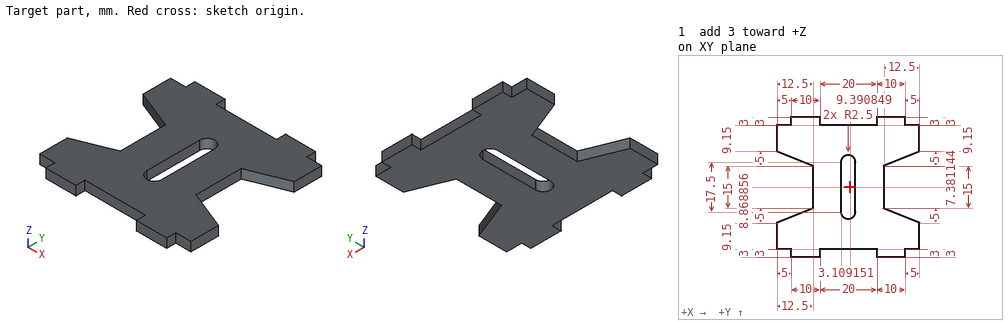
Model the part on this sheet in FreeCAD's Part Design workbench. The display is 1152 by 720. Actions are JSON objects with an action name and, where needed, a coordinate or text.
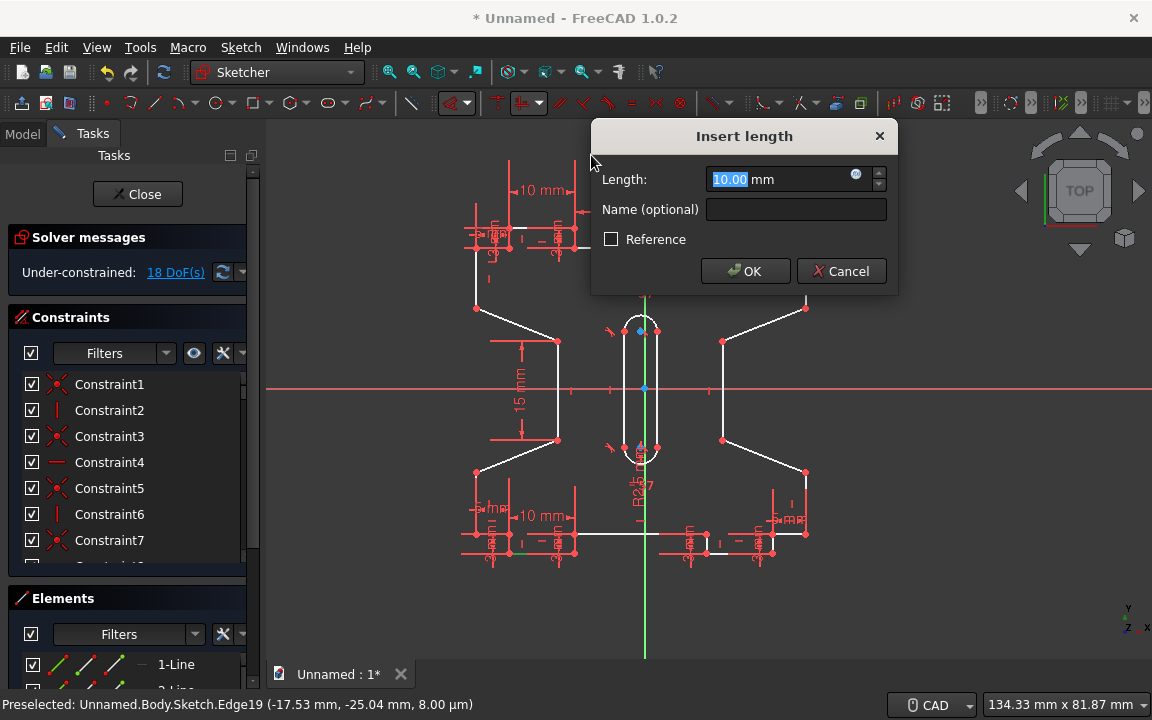
{"action": "type", "text": "10"}
{"action": "key", "text": "Return"}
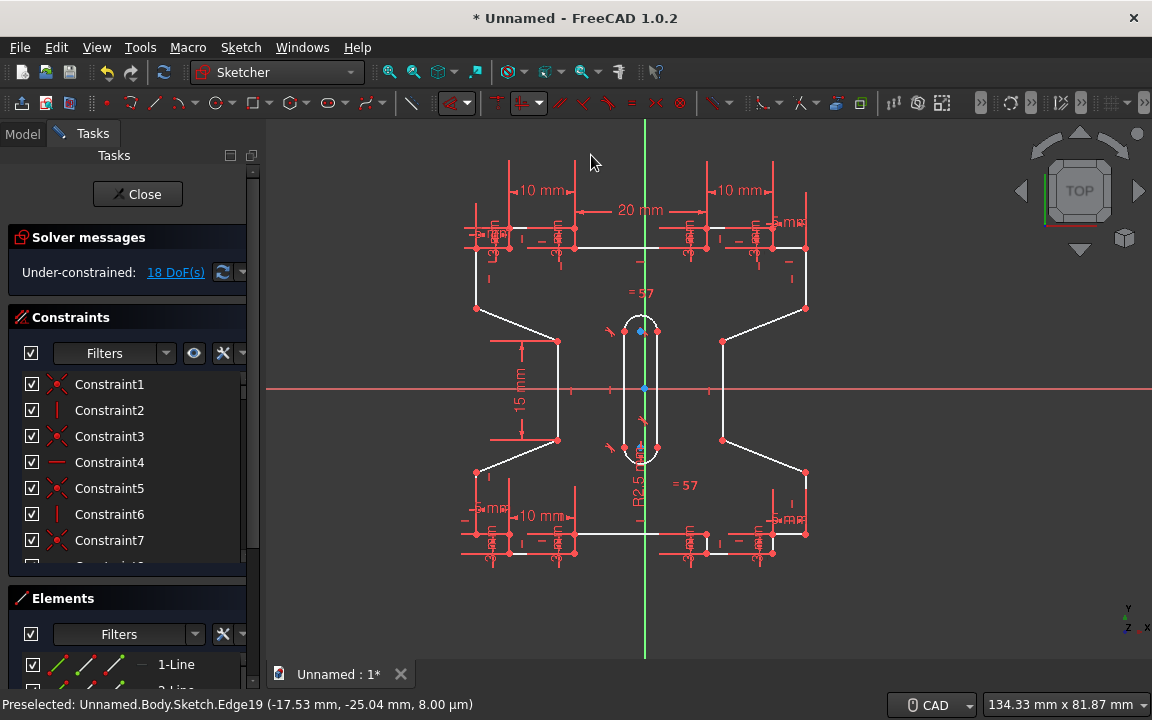
{"action": "left_click", "coordinate": [615, 534]}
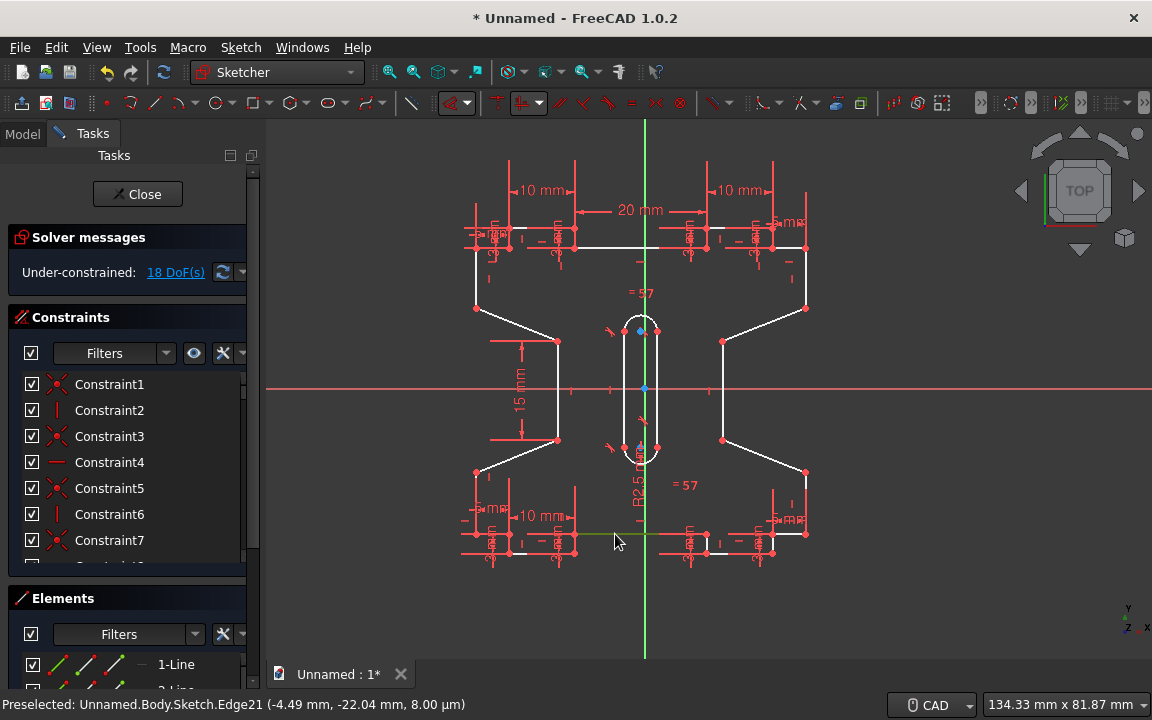
{"action": "key", "text": "l"}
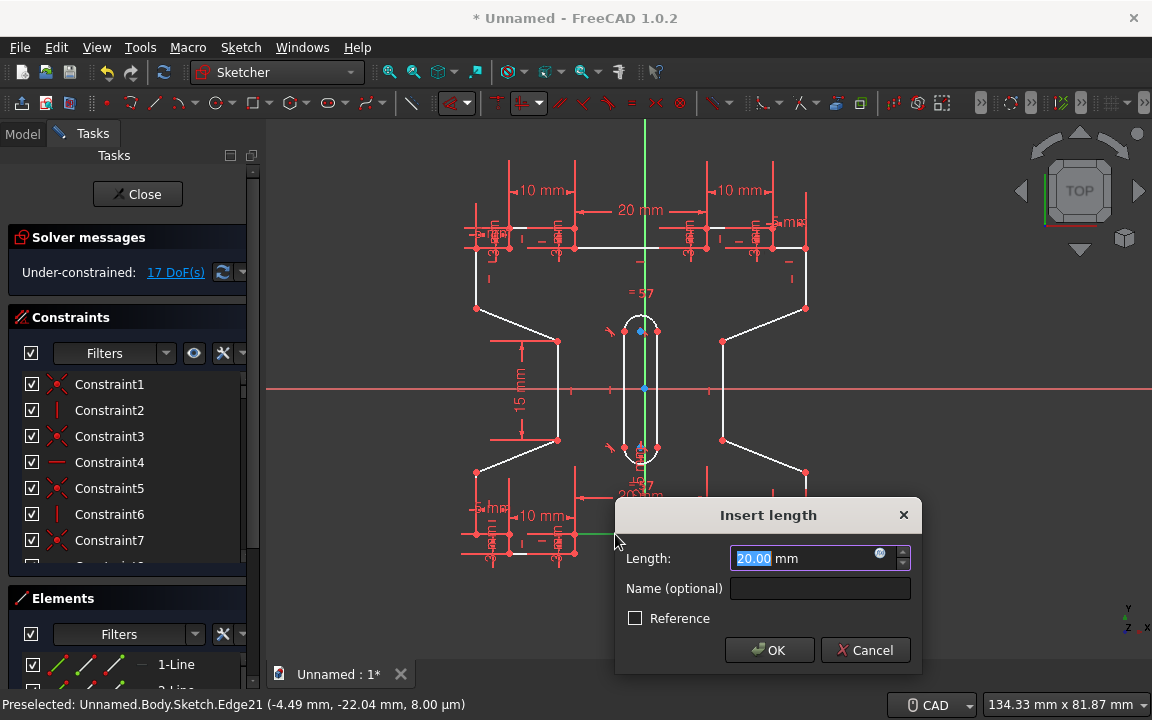
{"action": "type", "text": "20"}
{"action": "key", "text": "Return"}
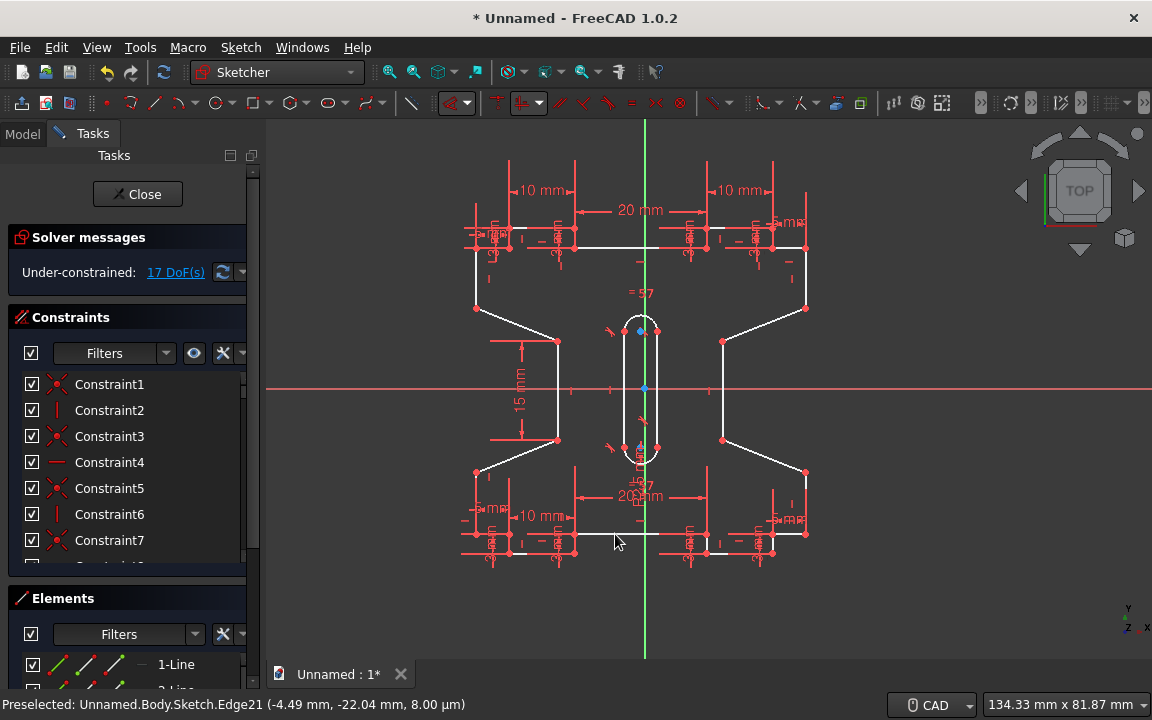
{"action": "left_click", "coordinate": [727, 554]}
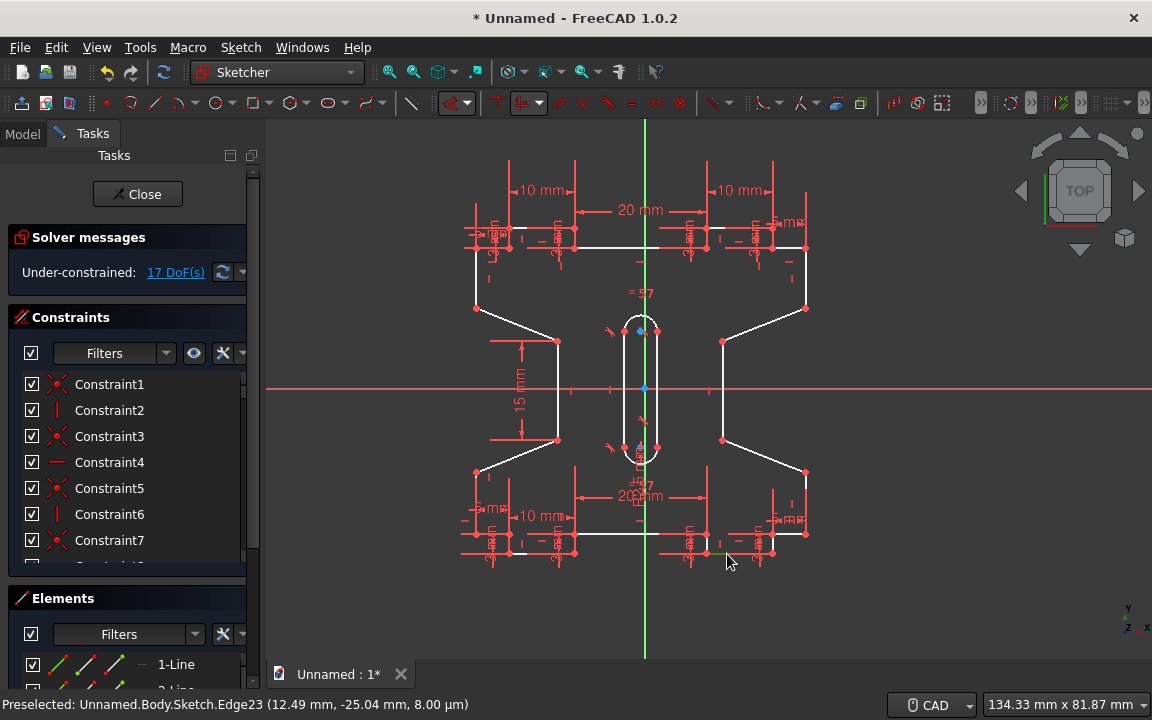
{"action": "left_click", "coordinate": [470, 104]}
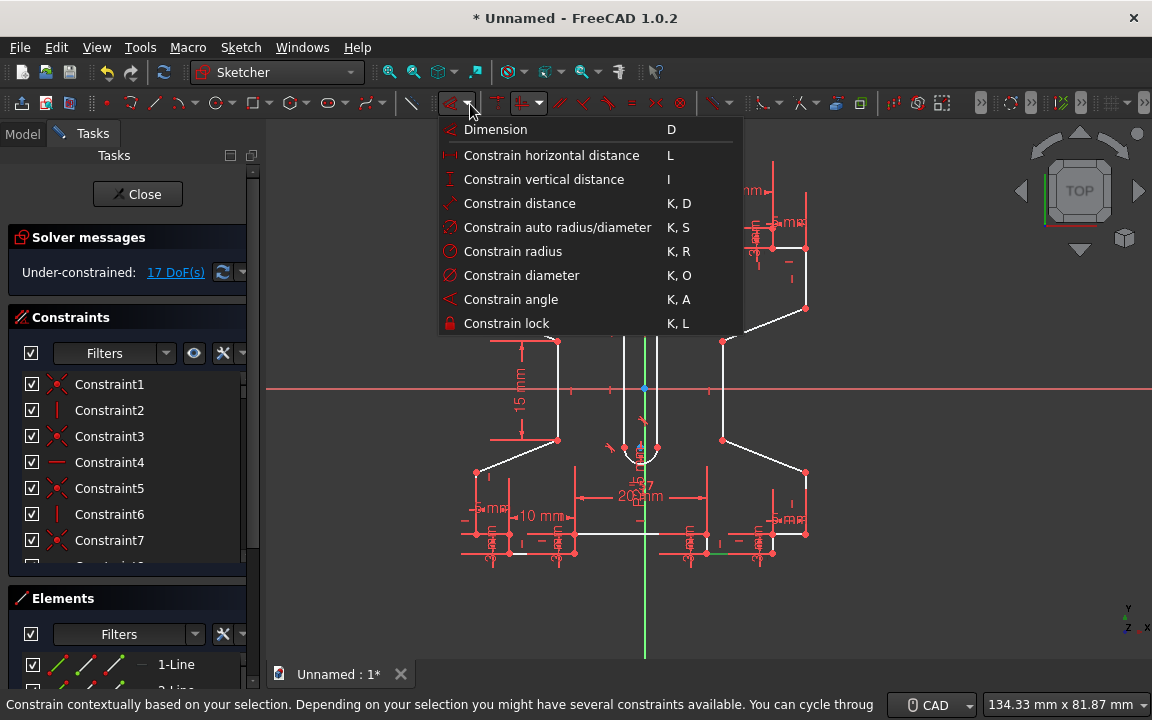
{"action": "left_click", "coordinate": [591, 155]}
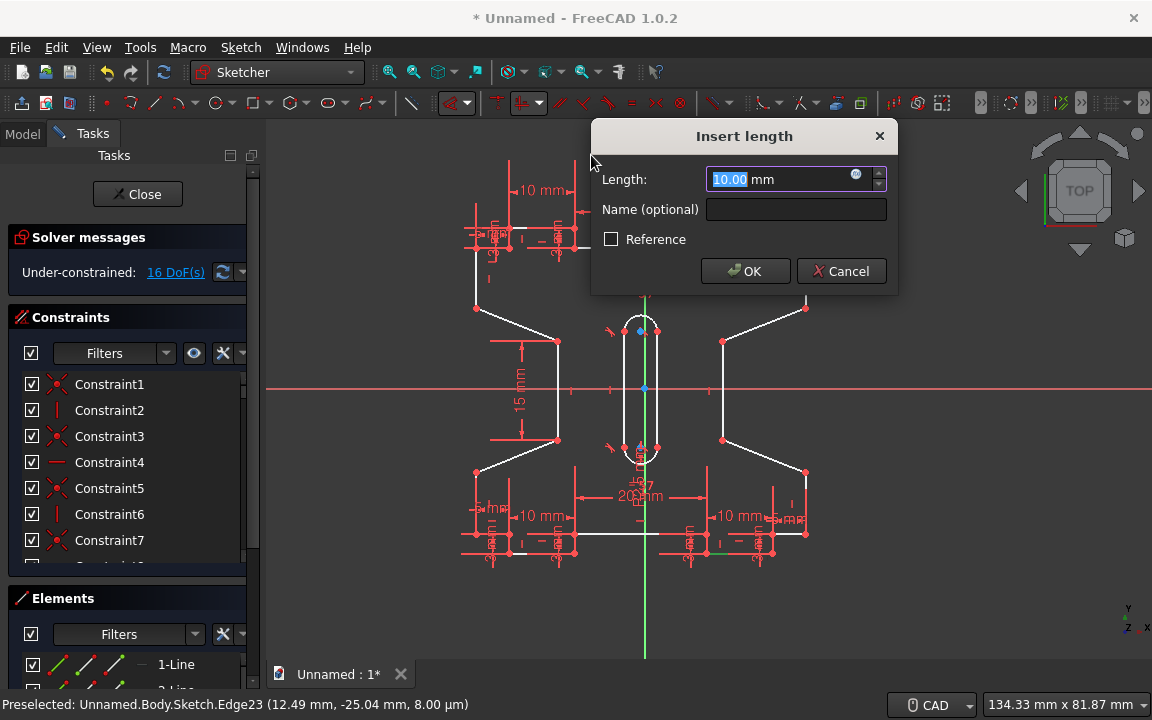
{"action": "type", "text": "10"}
{"action": "key", "text": "Return"}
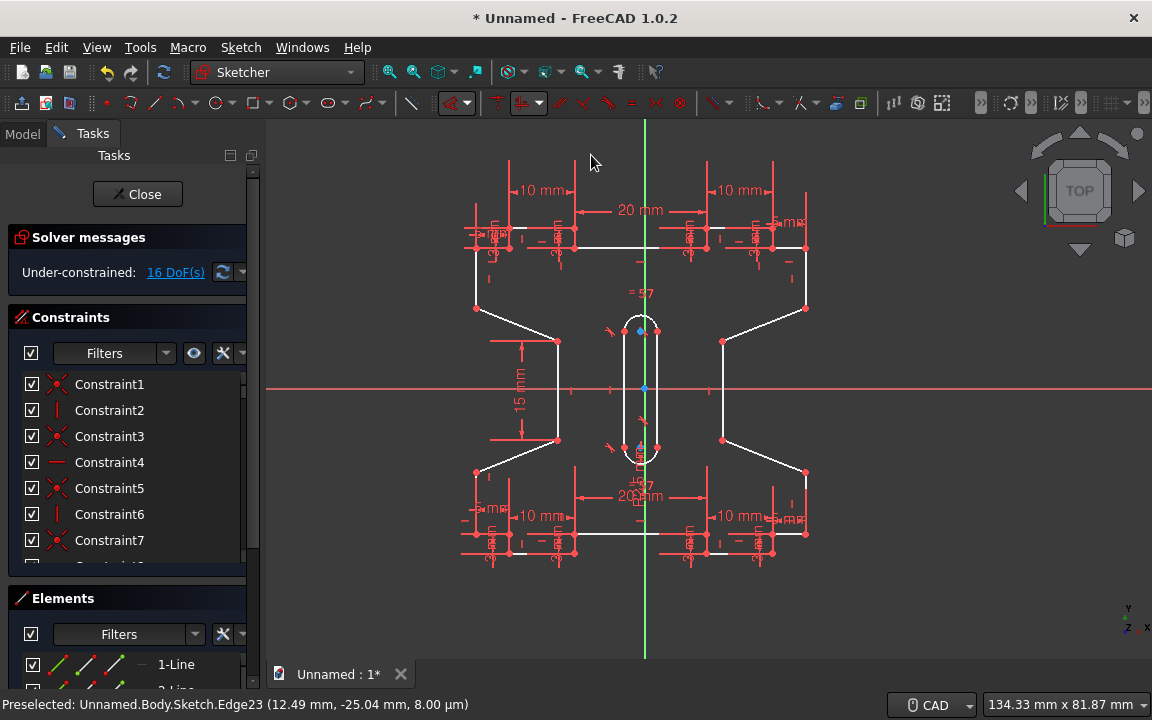
{"action": "left_click", "coordinate": [723, 410]}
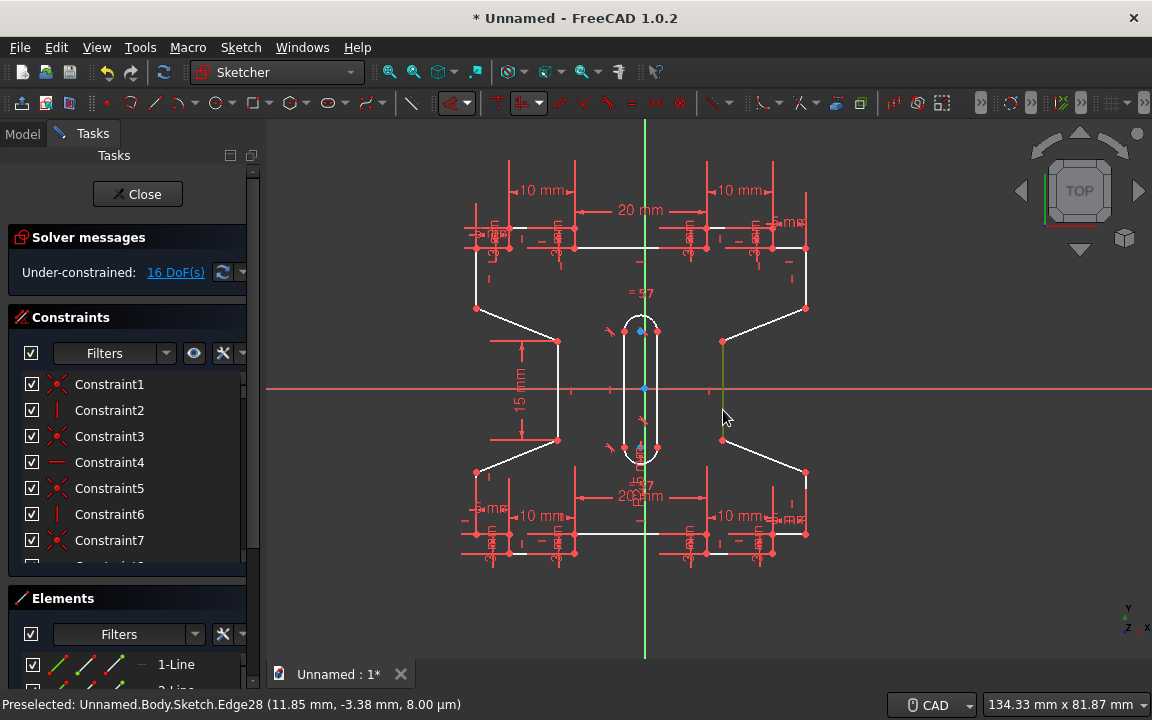
{"action": "left_click", "coordinate": [470, 104]}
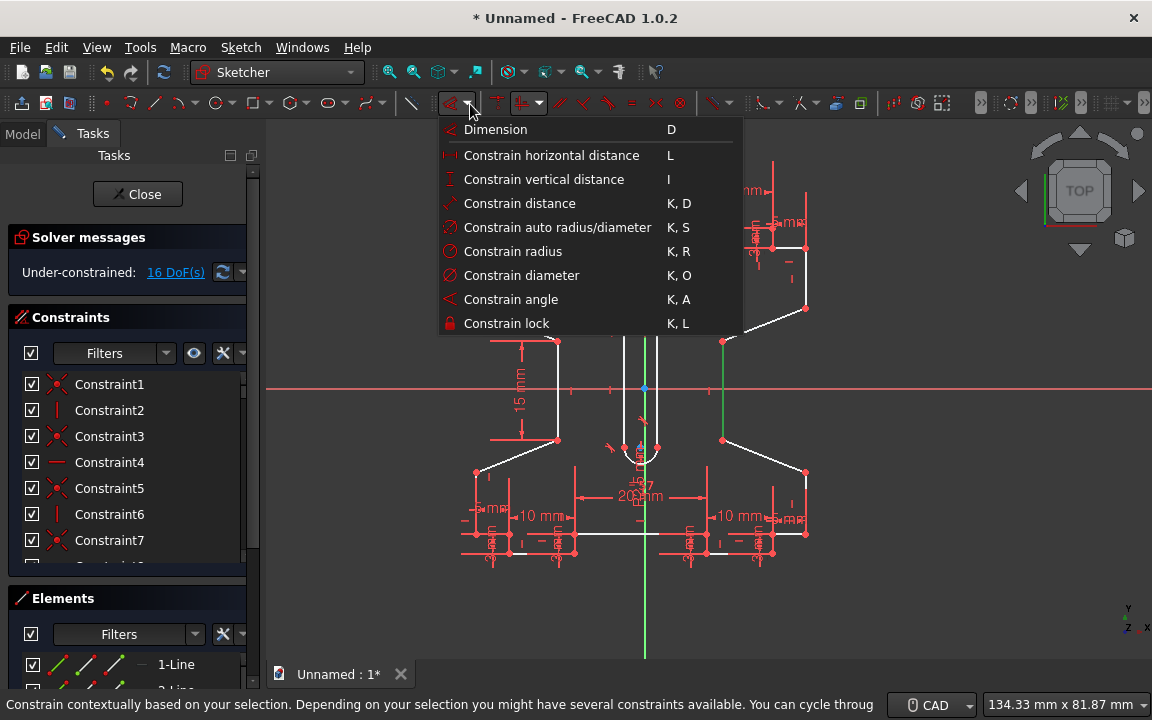
{"action": "left_click", "coordinate": [591, 179]}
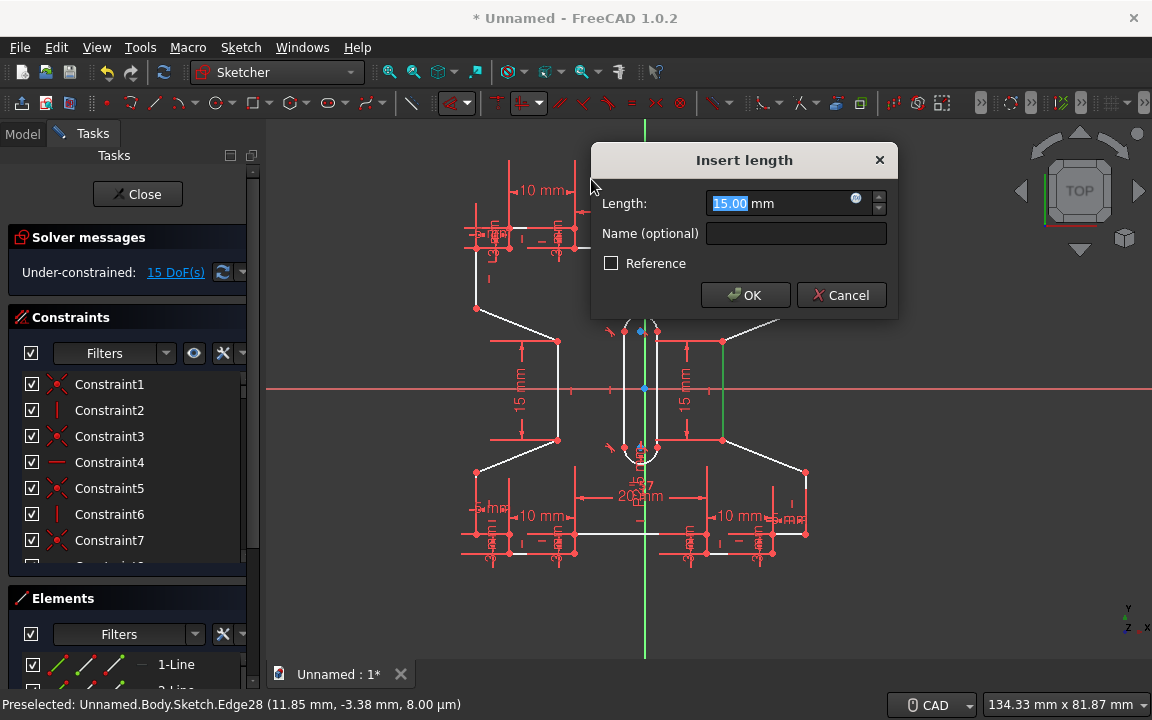
{"action": "type", "text": "15"}
{"action": "key", "text": "Return"}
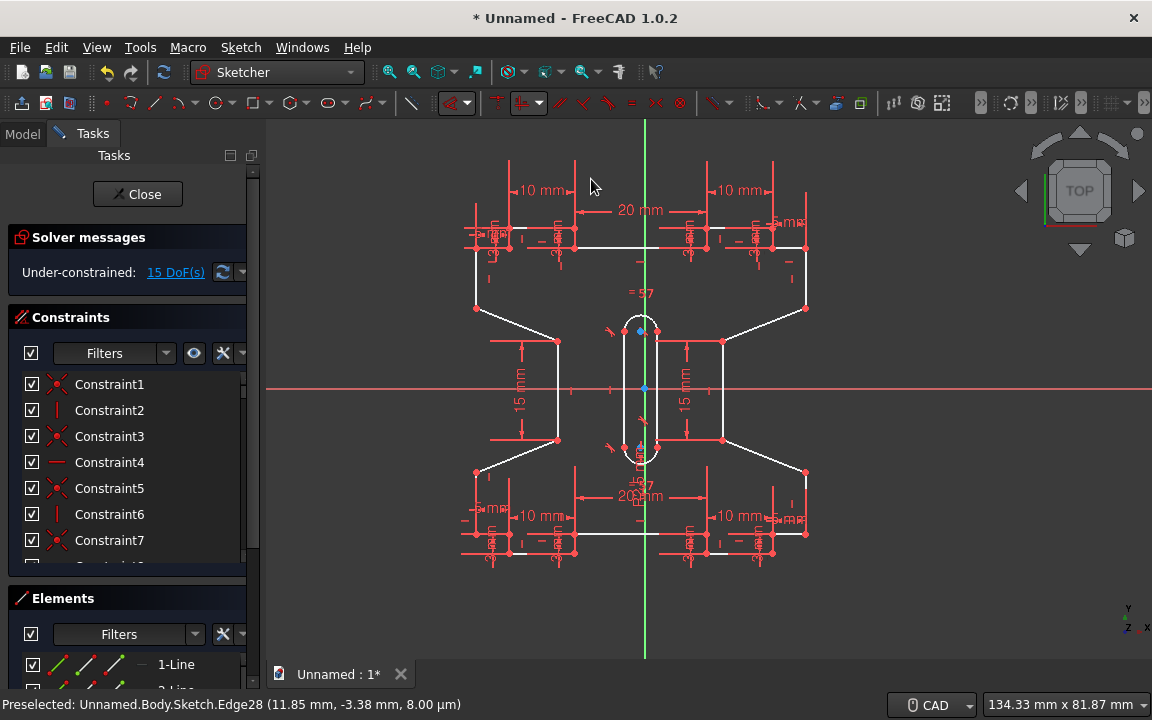
{"action": "left_click", "coordinate": [748, 331]}